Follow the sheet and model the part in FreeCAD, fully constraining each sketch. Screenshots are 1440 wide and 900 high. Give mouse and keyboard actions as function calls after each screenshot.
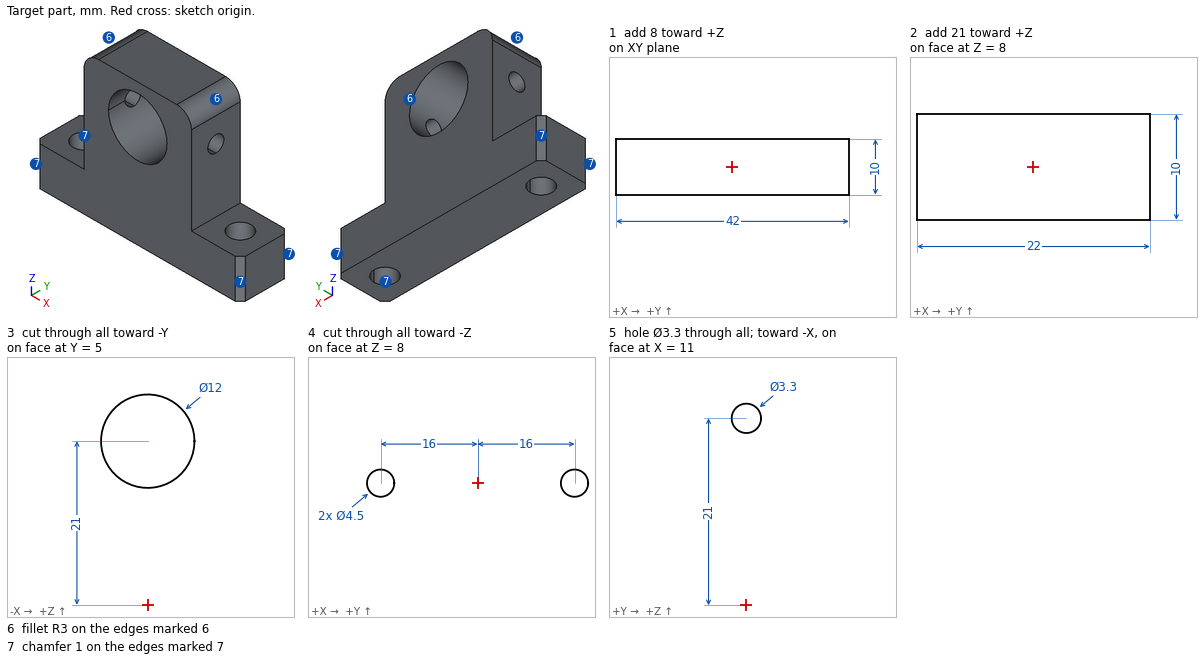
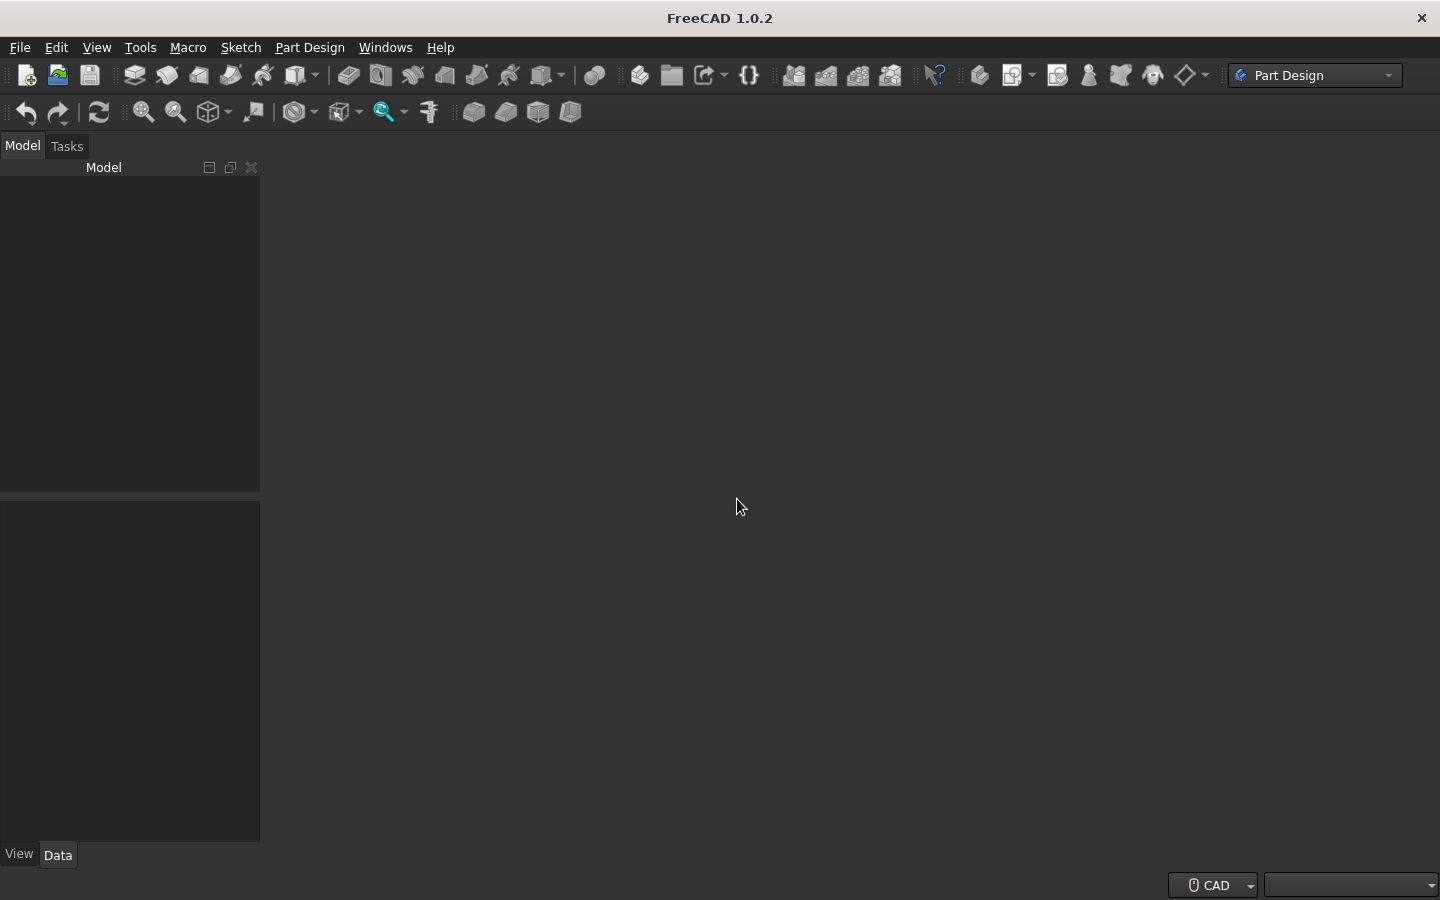
click(26, 76)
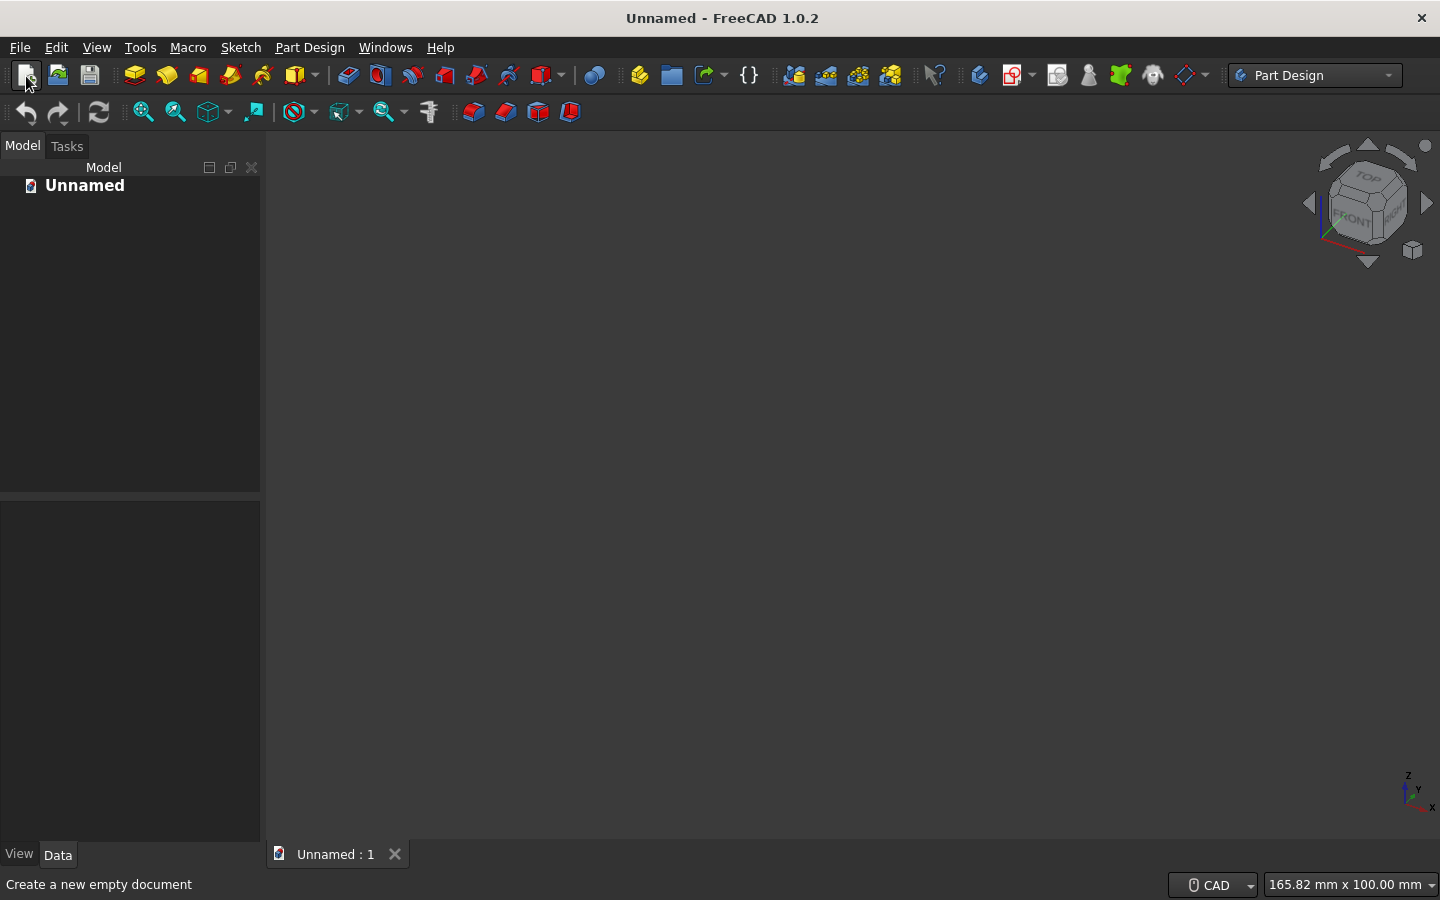
click(1012, 76)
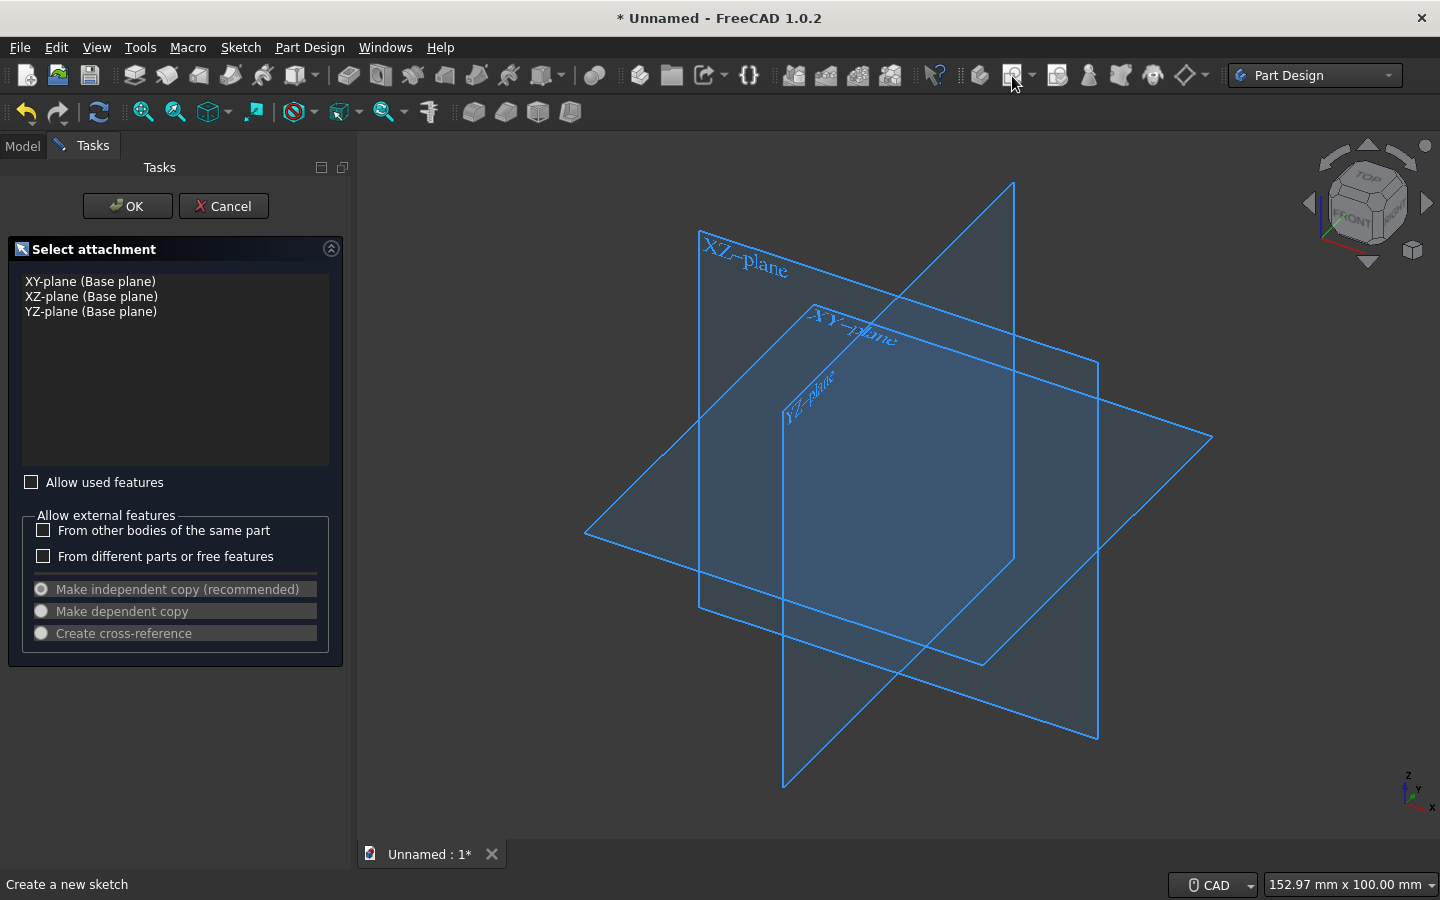
click(82, 282)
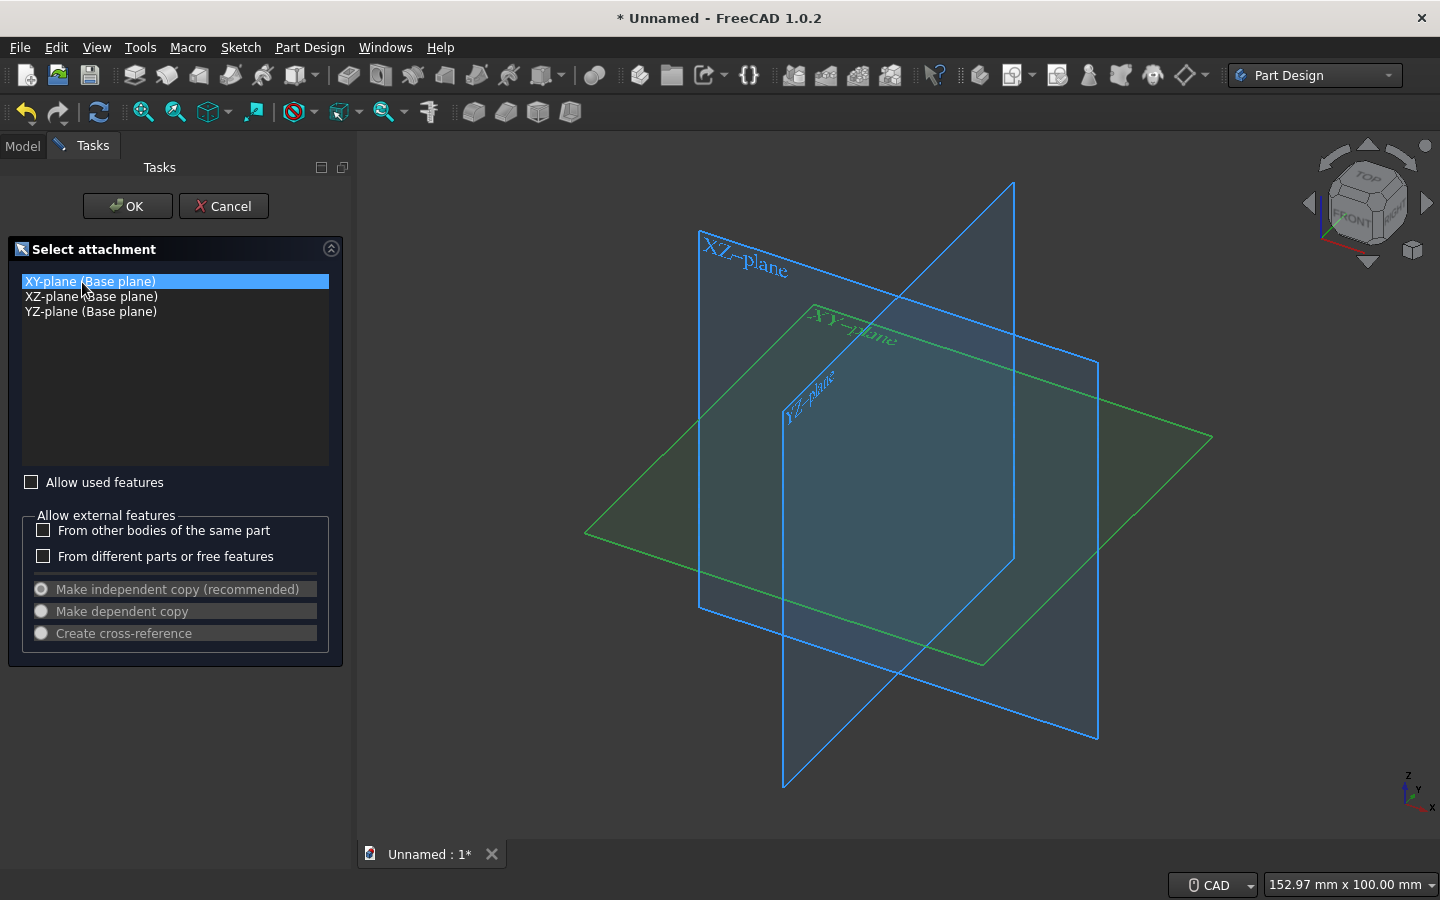
click(128, 206)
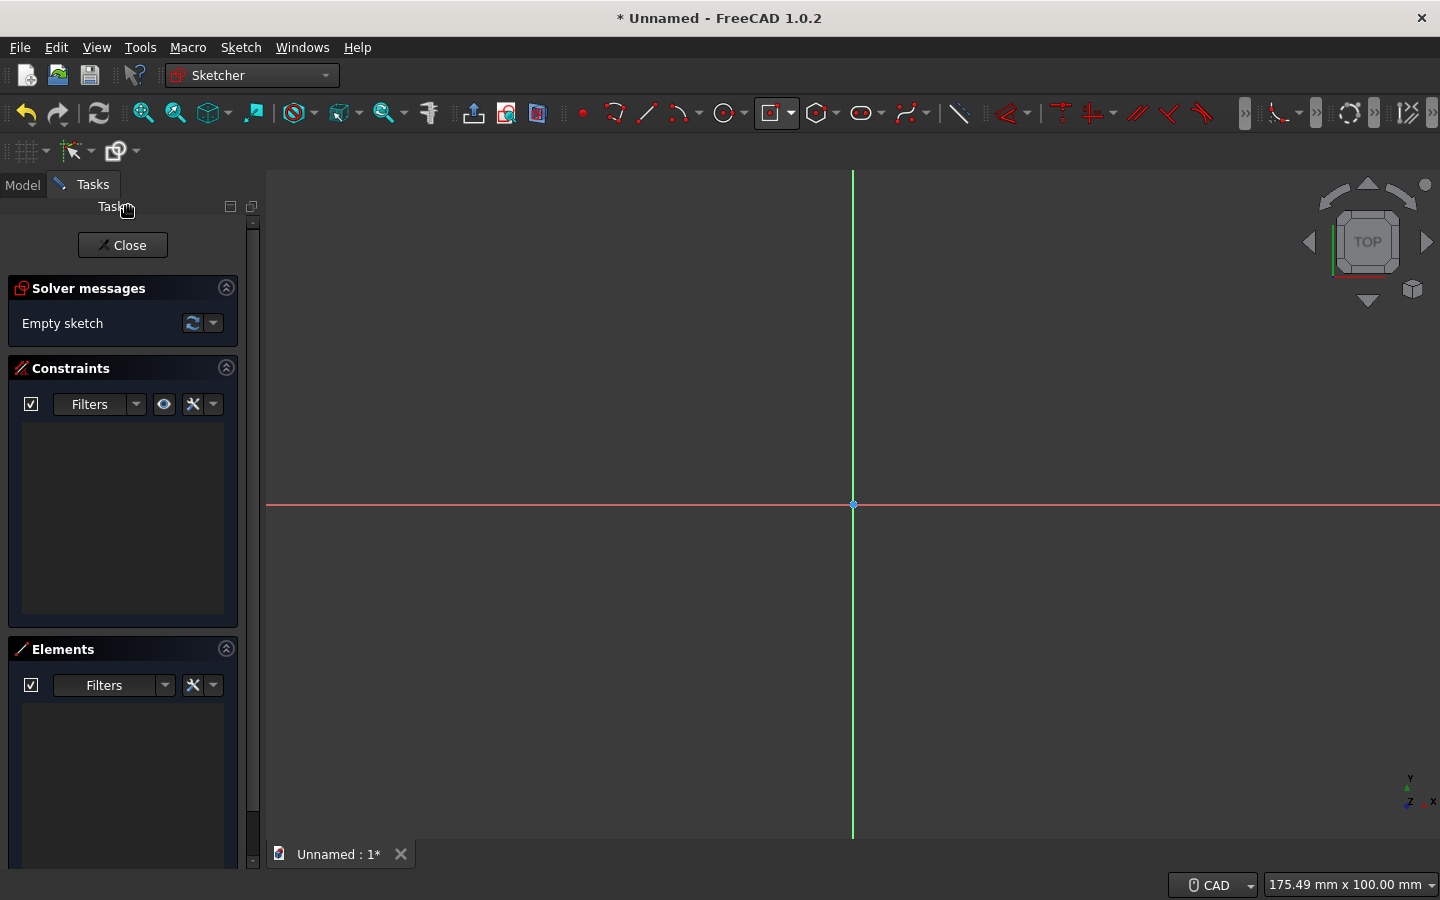
scroll(893, 504, up, 5)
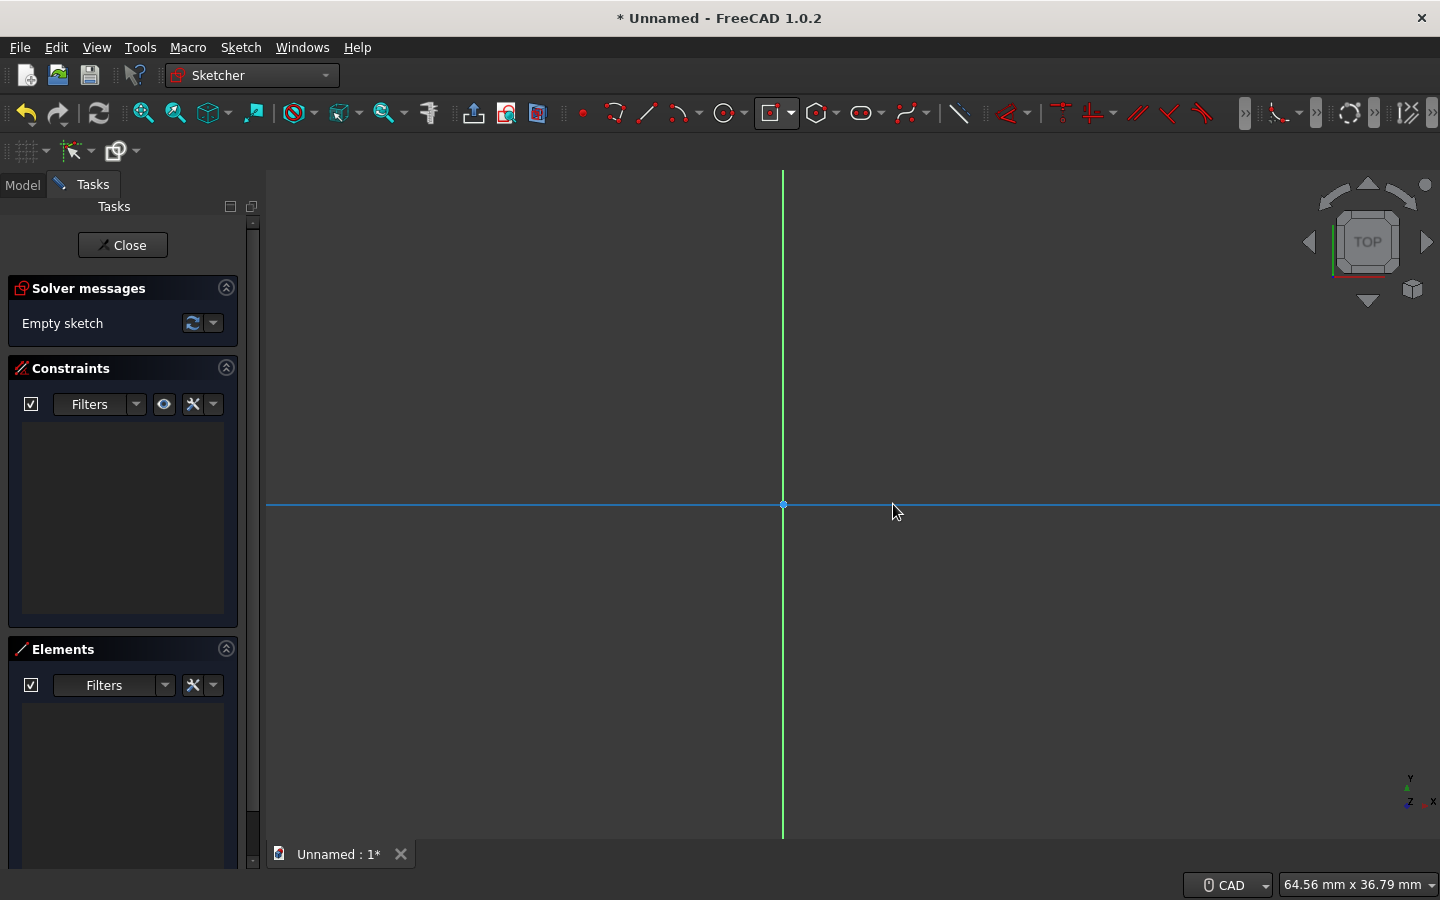
click(770, 114)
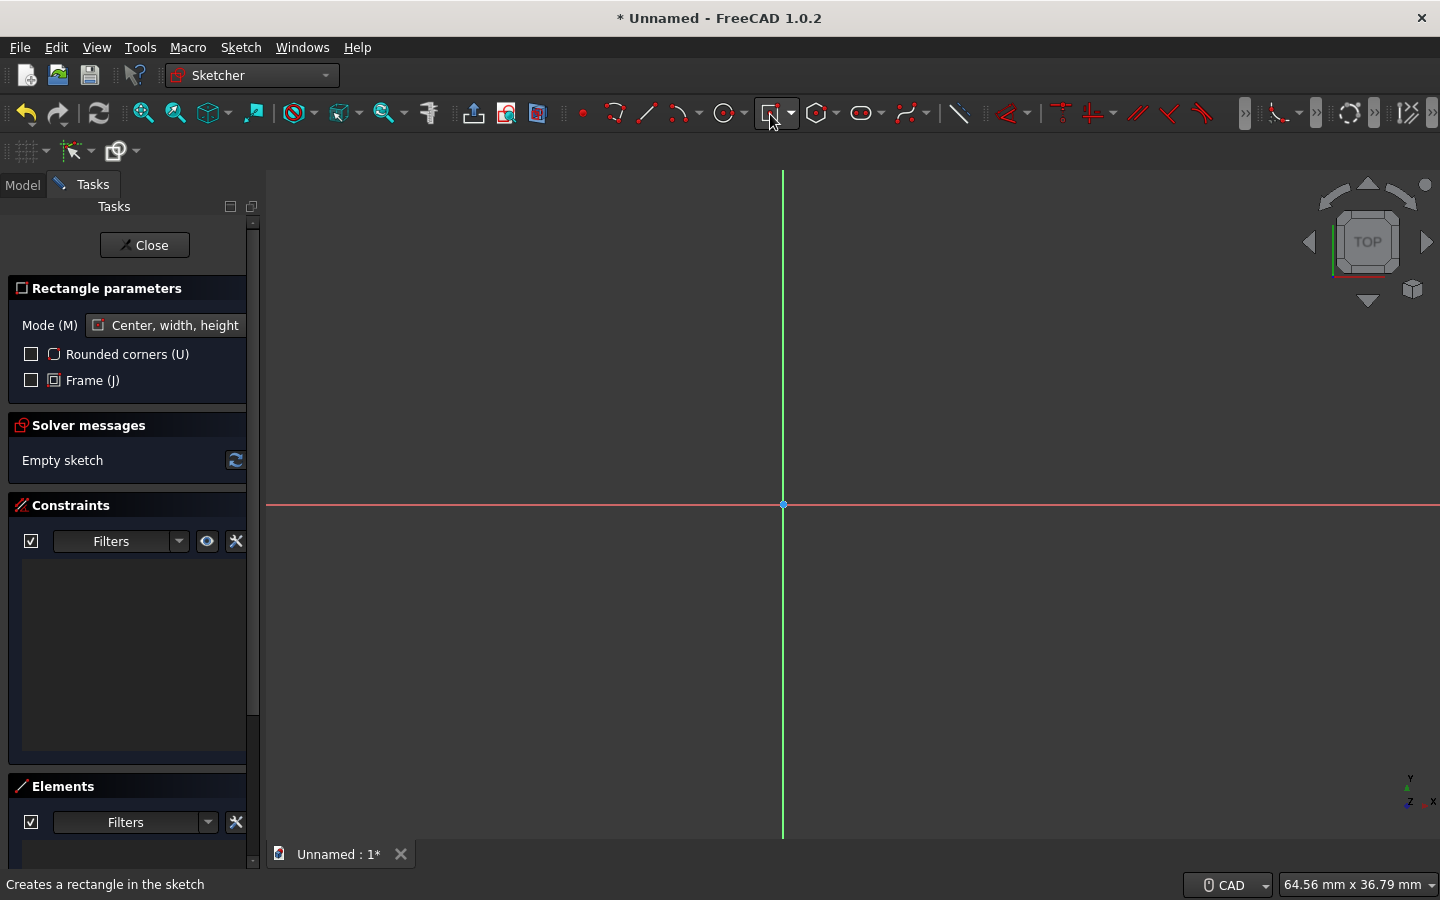
click(783, 504)
click(1165, 414)
key(Escape)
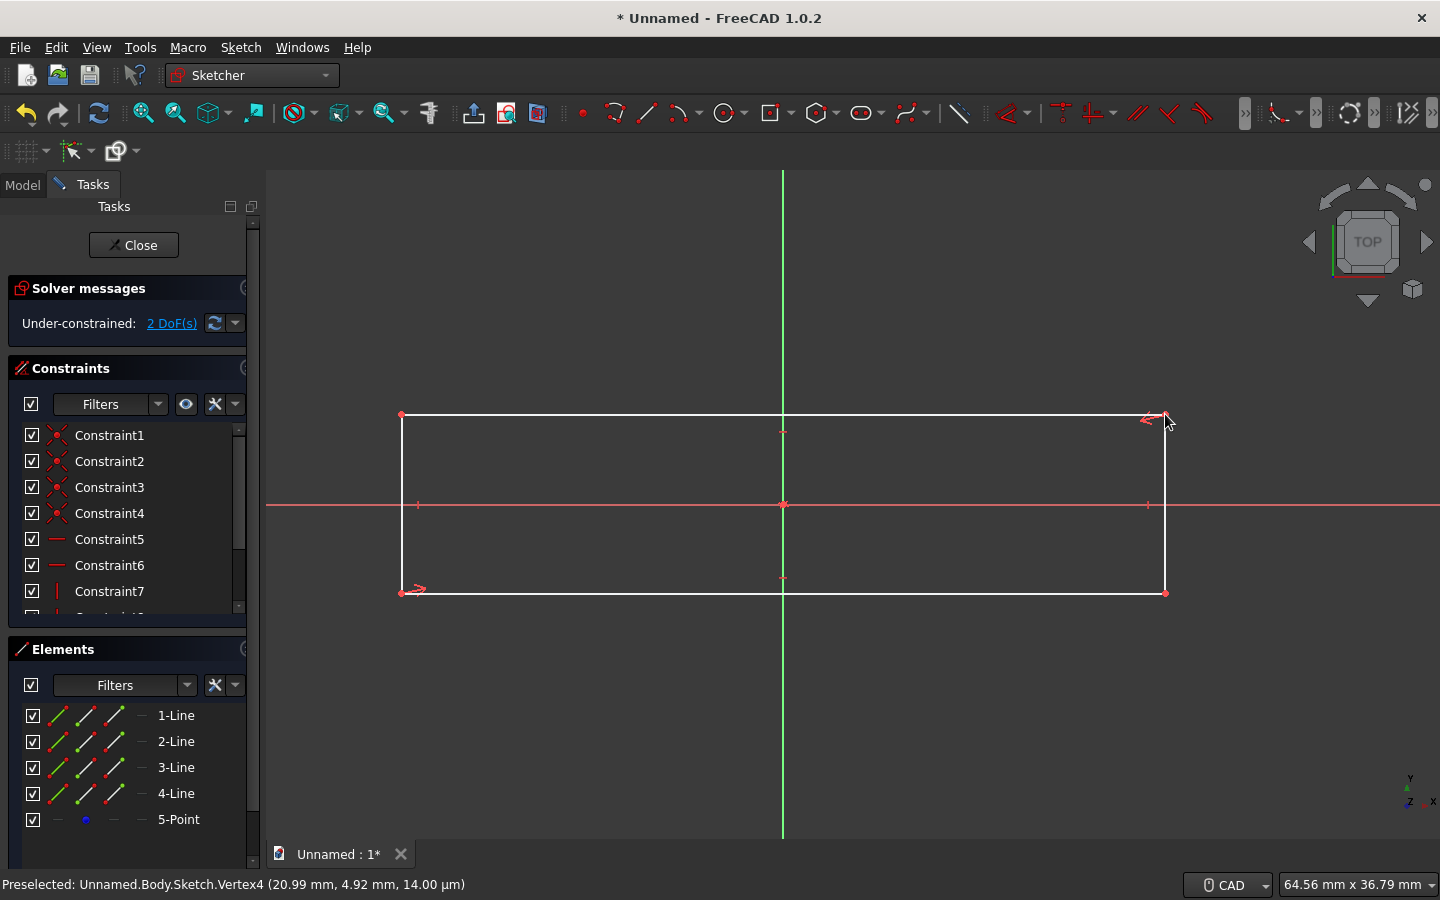
key(d)